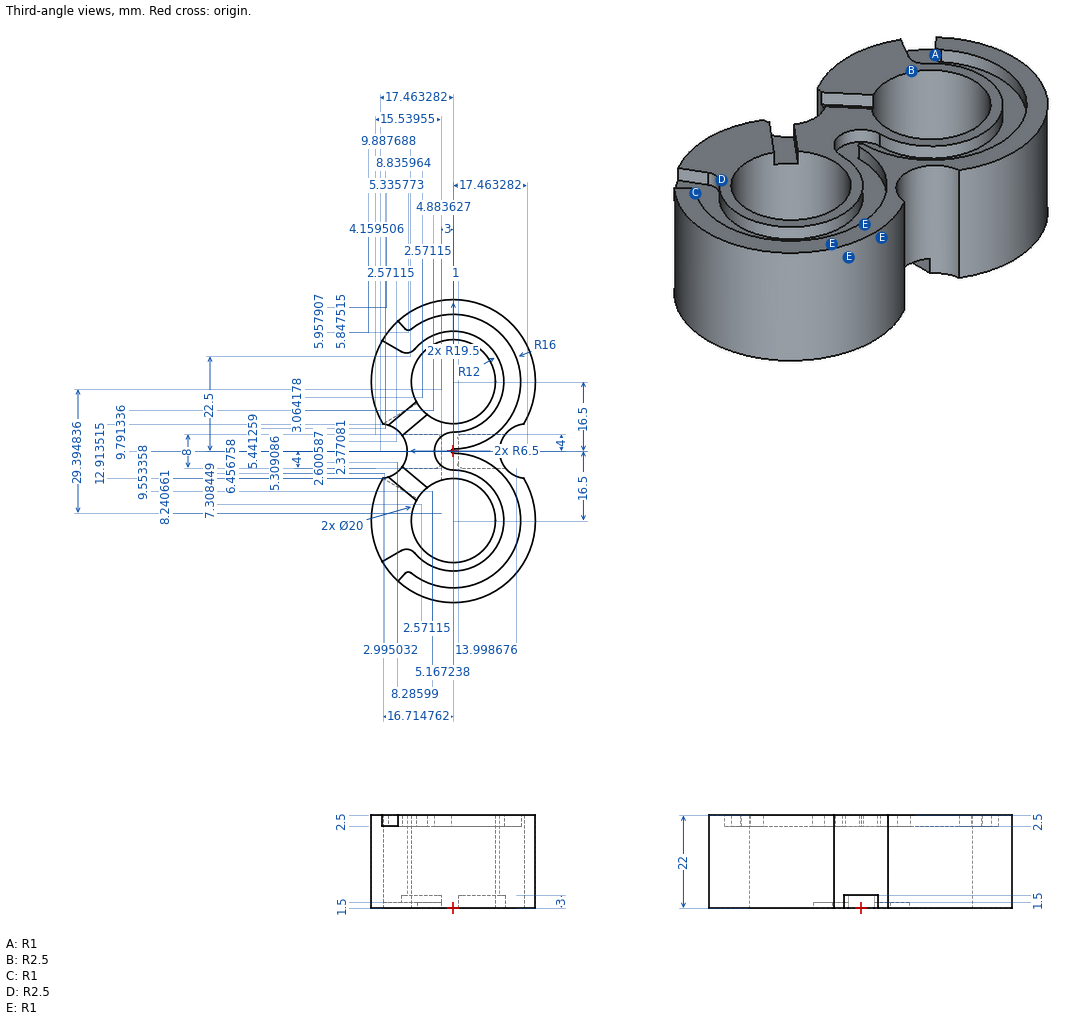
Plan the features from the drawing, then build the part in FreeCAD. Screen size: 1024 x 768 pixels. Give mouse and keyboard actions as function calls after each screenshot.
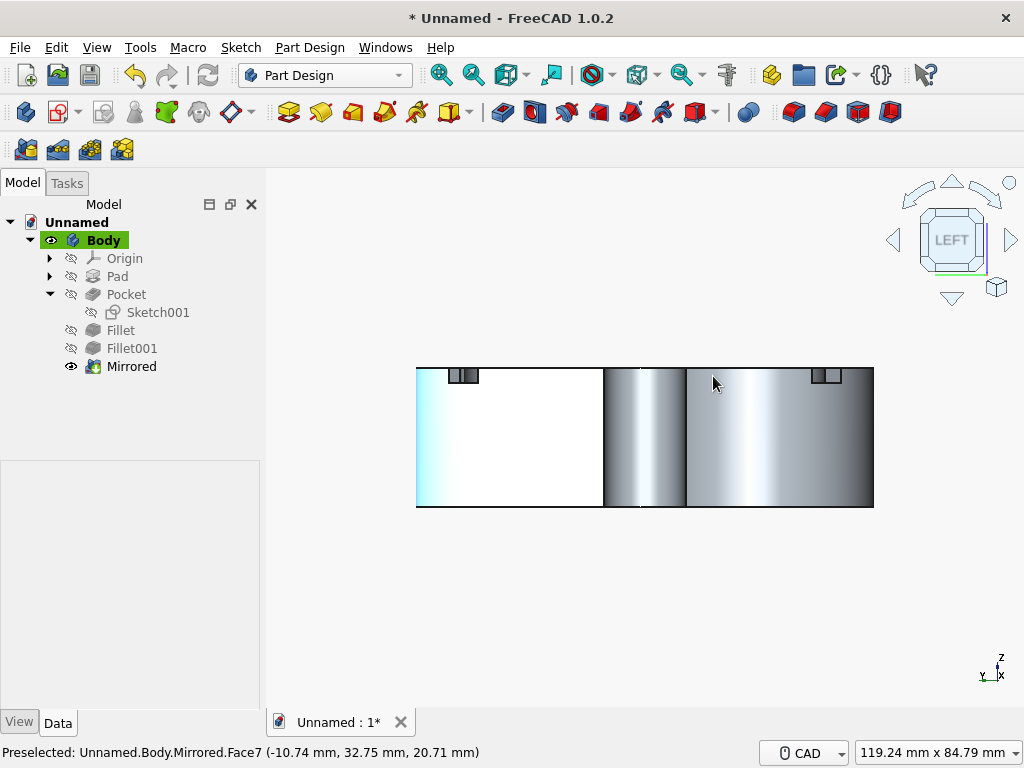
scroll(825, 375, up, 5)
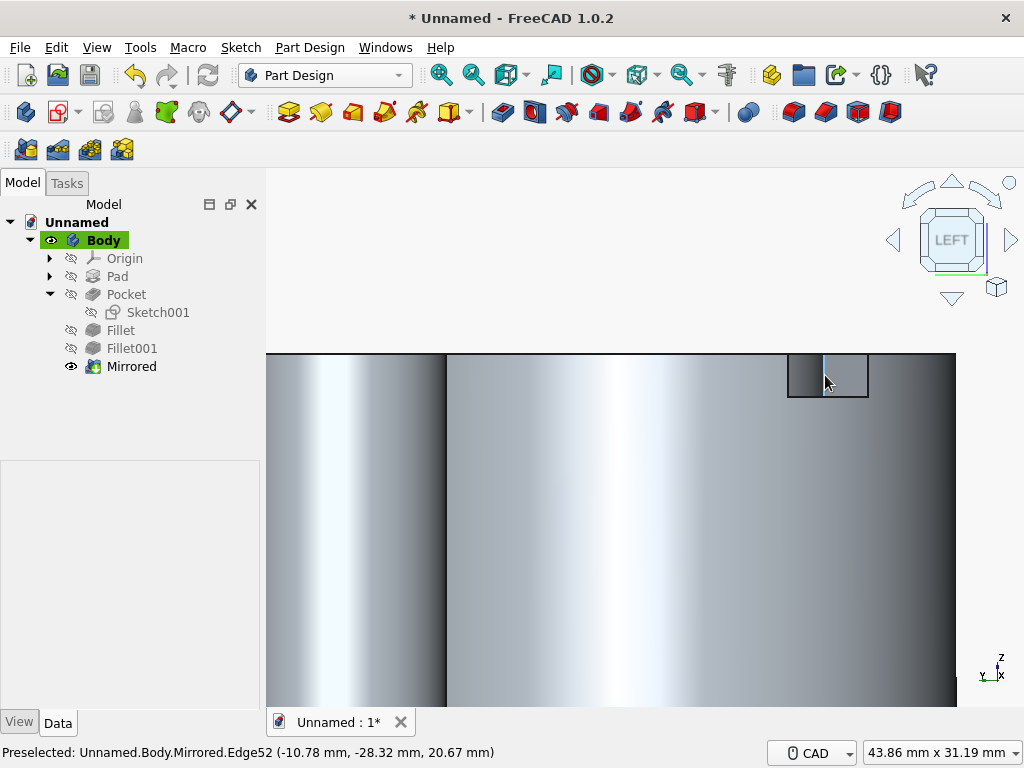
click(442, 76)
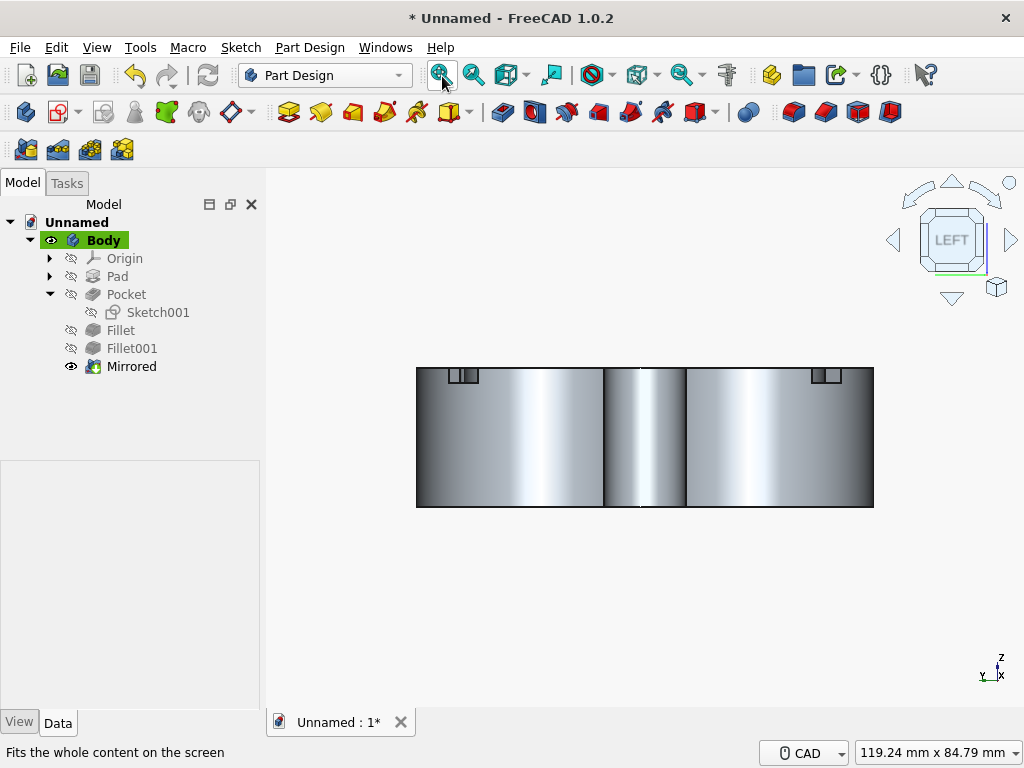
key(v)
key(3)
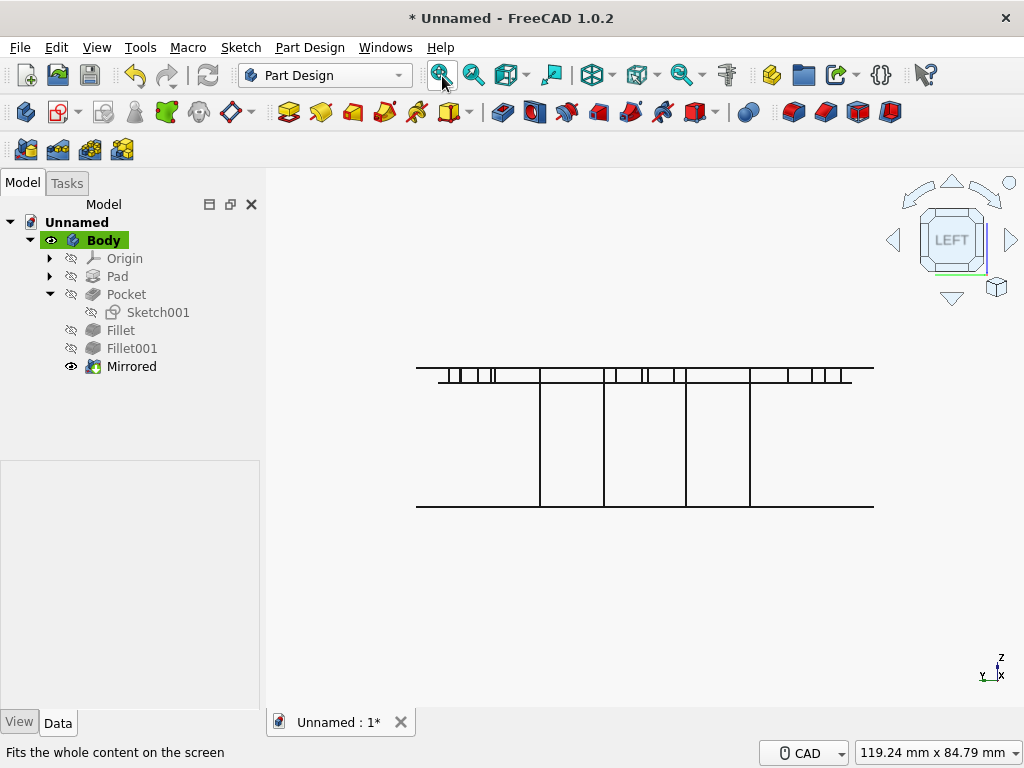
key(0)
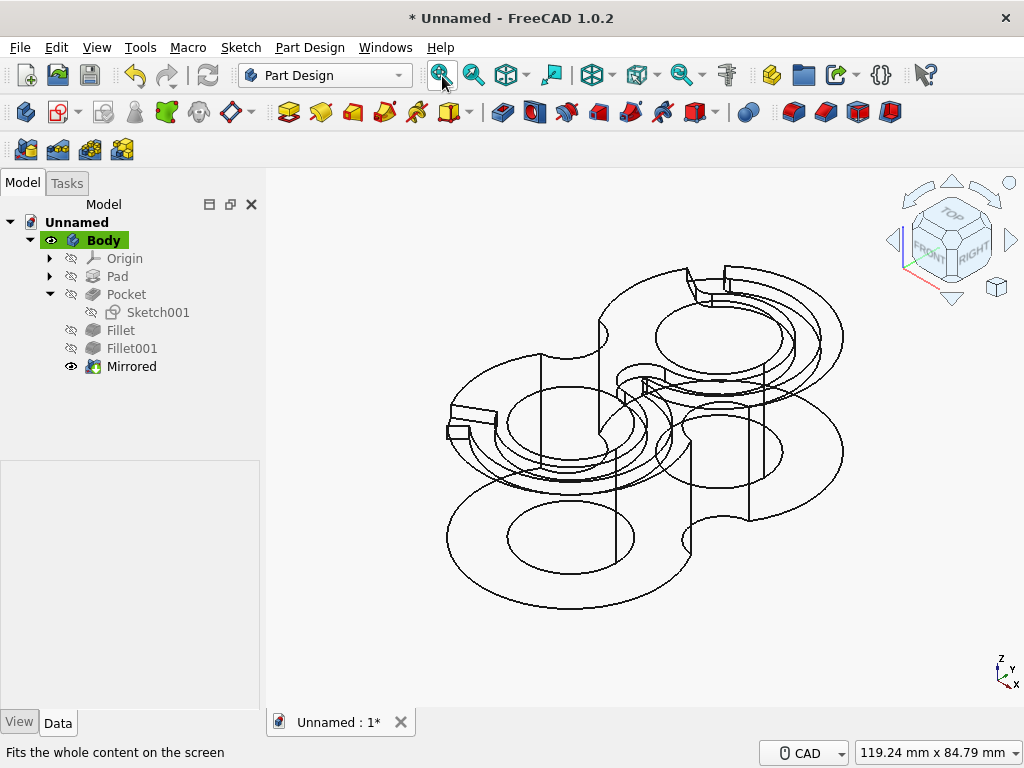
scroll(469, 431, up, 6)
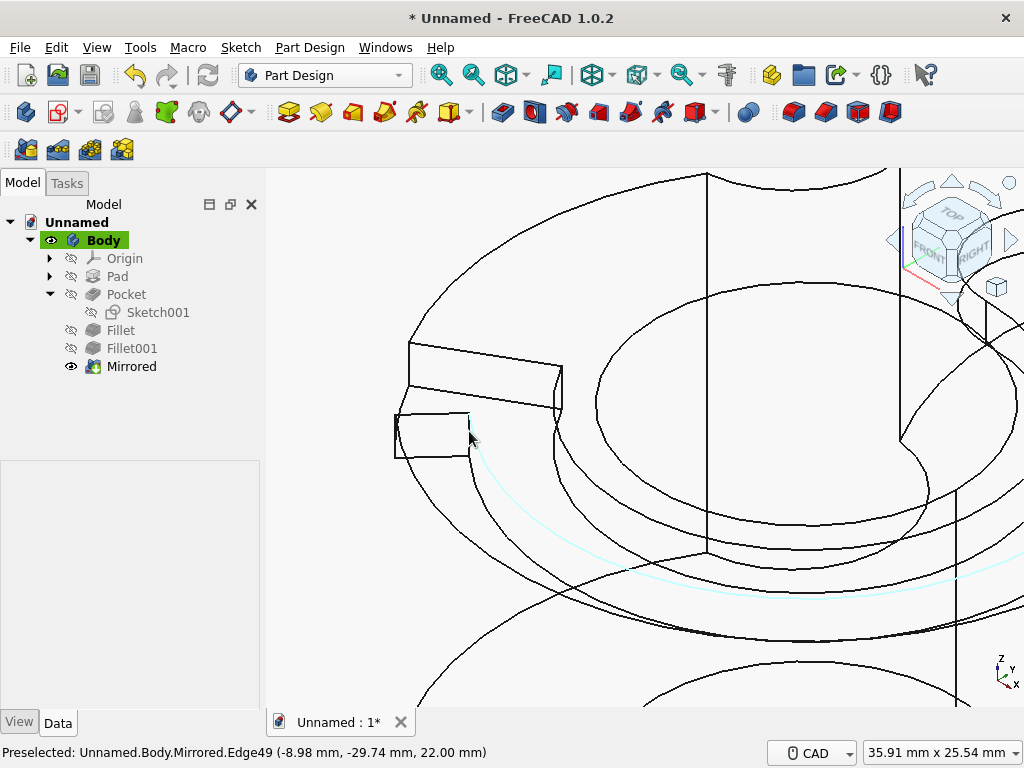
click(469, 446)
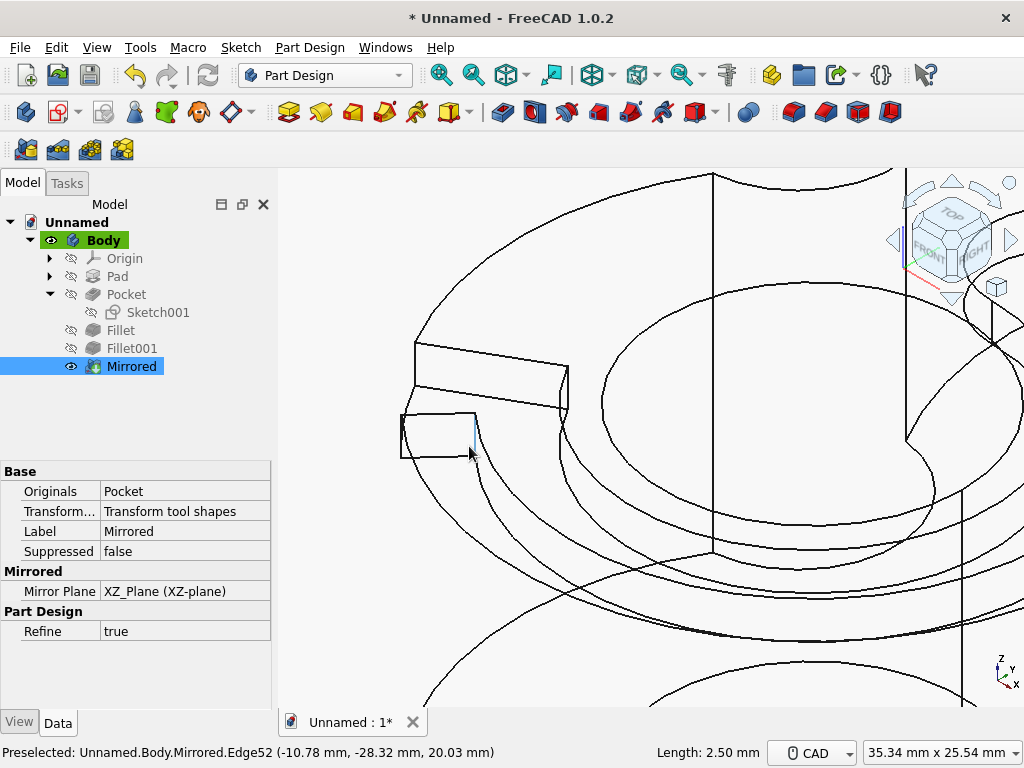
key(v)
key(1)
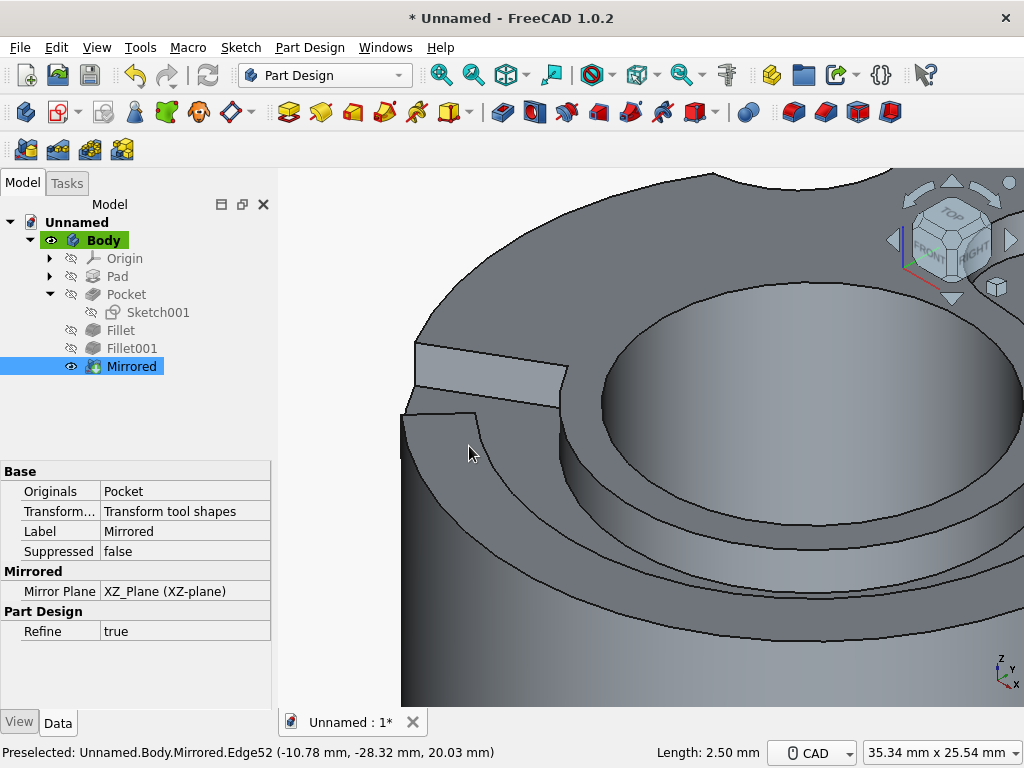
click(794, 112)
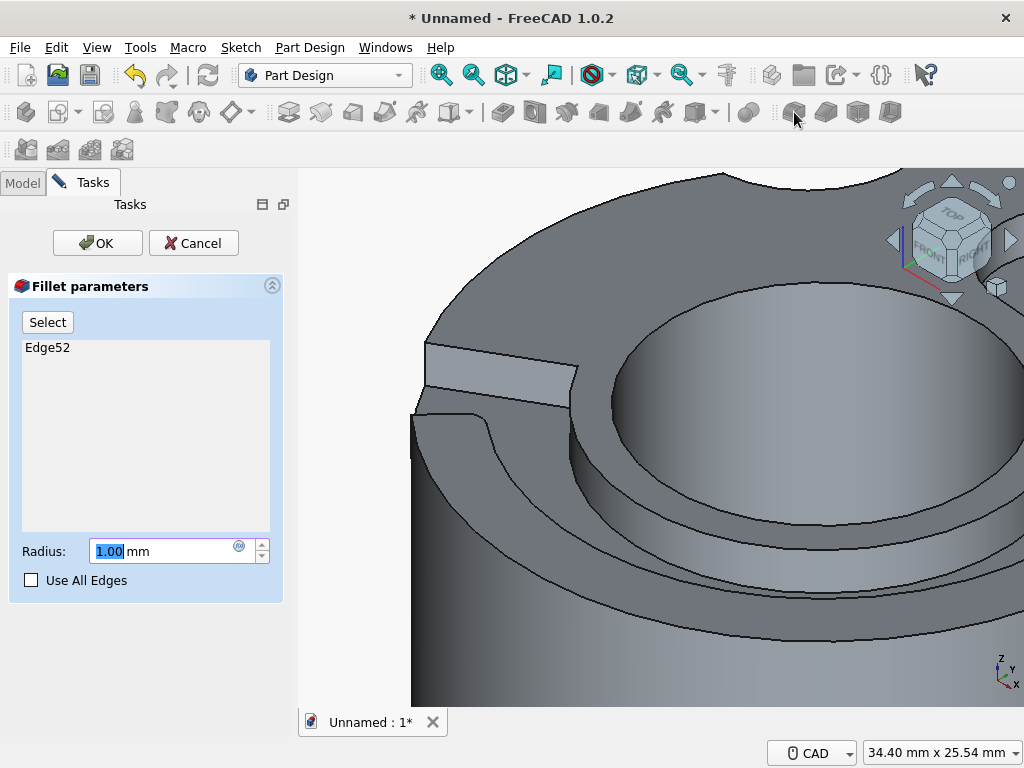
text(1)
key(Tab)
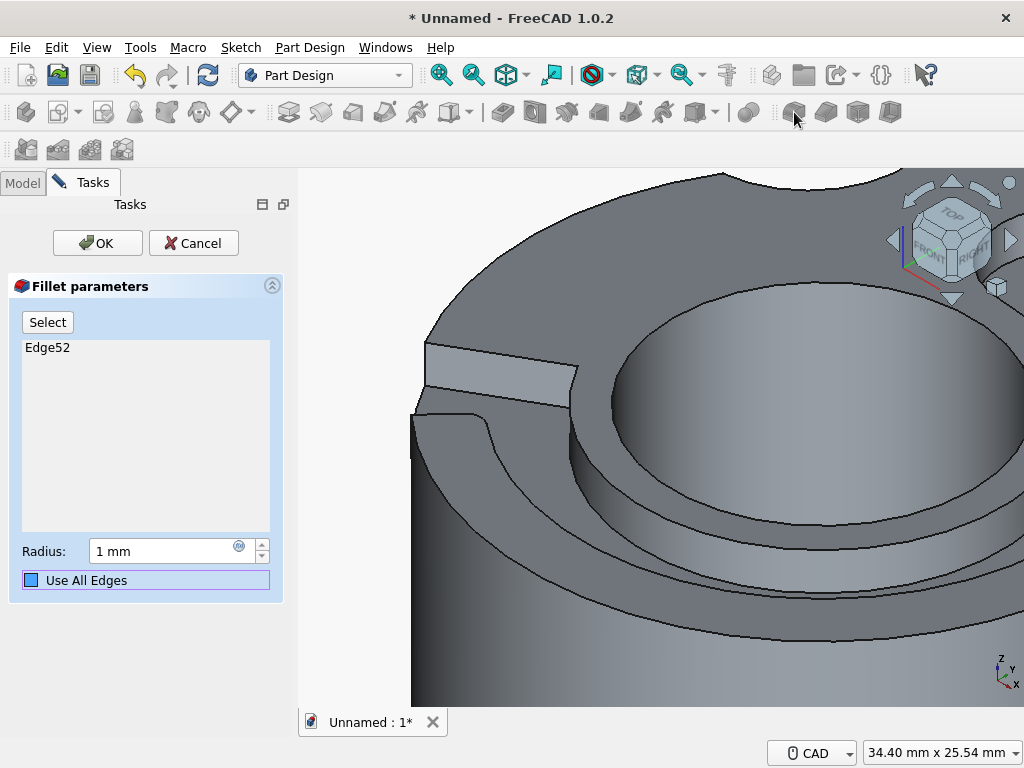
click(98, 243)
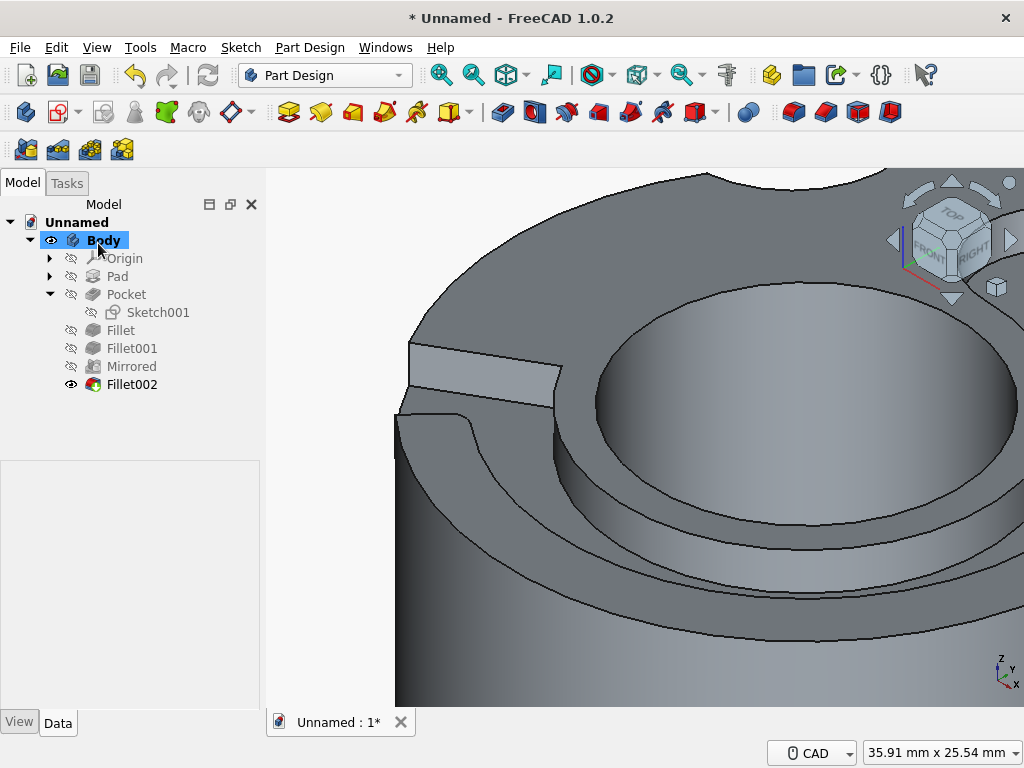
click(442, 76)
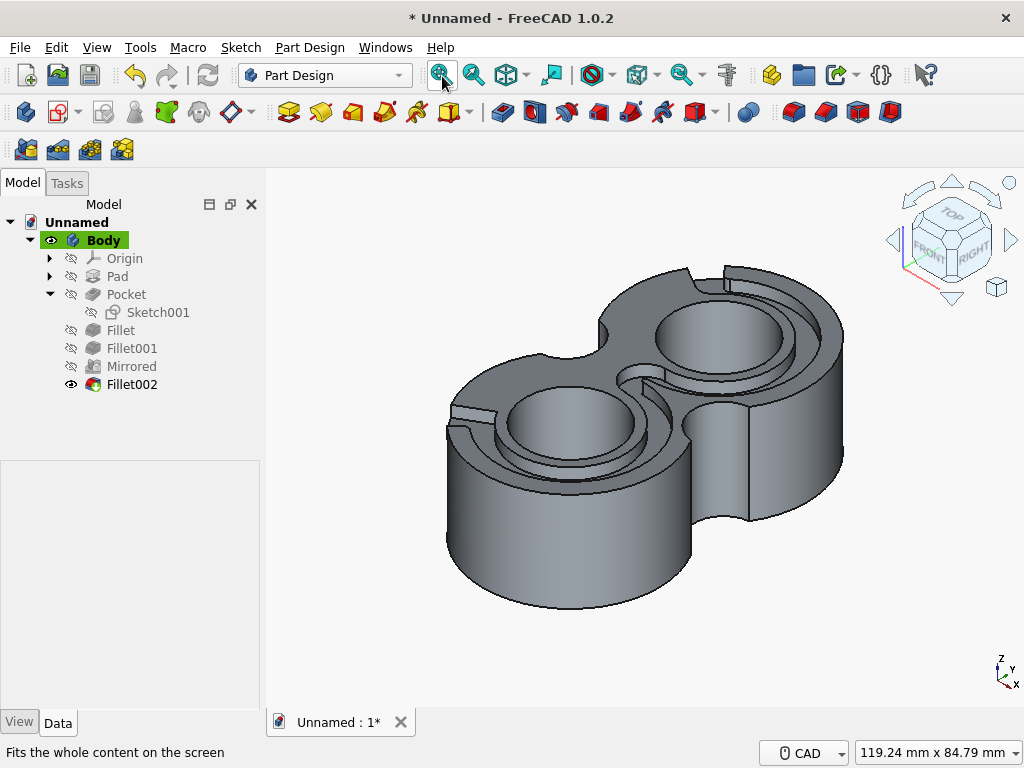
scroll(497, 417, up, 5)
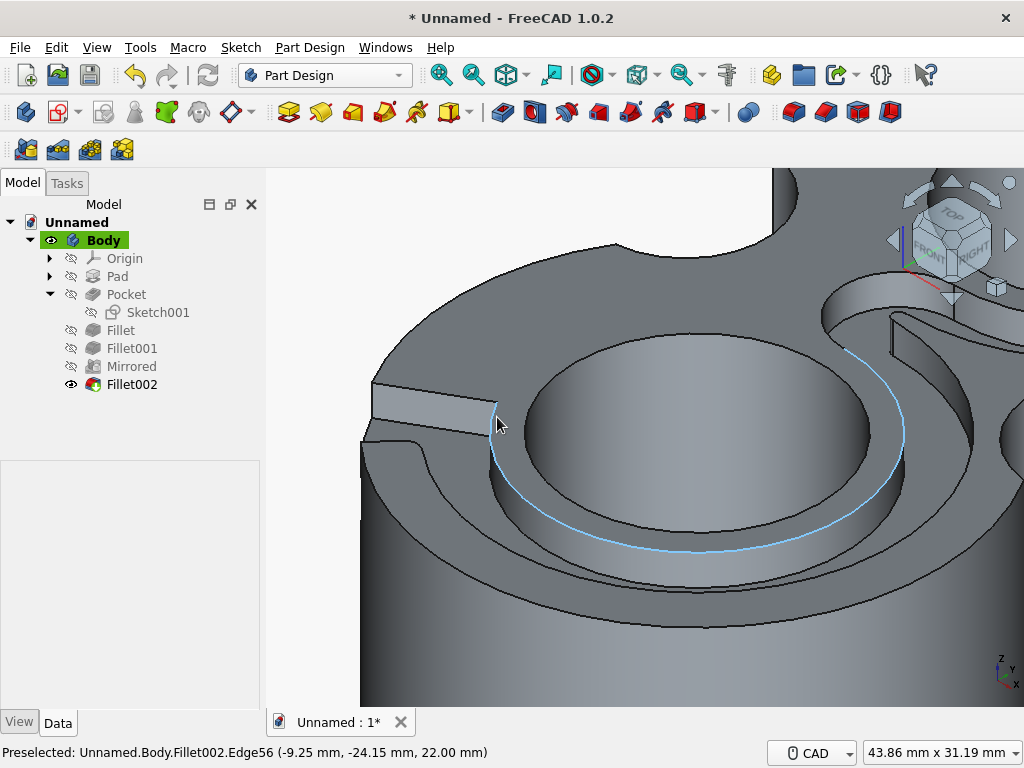
key(v)
key(f)